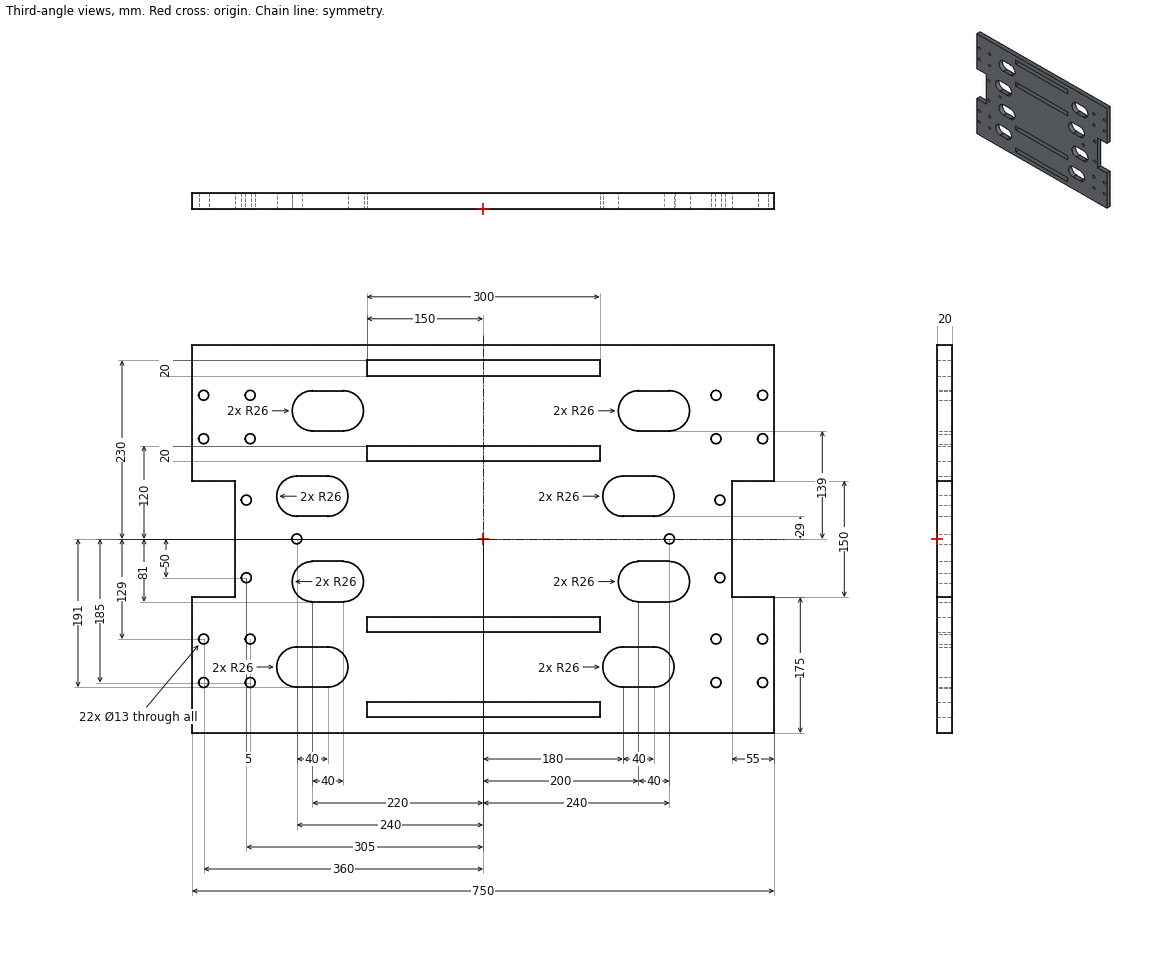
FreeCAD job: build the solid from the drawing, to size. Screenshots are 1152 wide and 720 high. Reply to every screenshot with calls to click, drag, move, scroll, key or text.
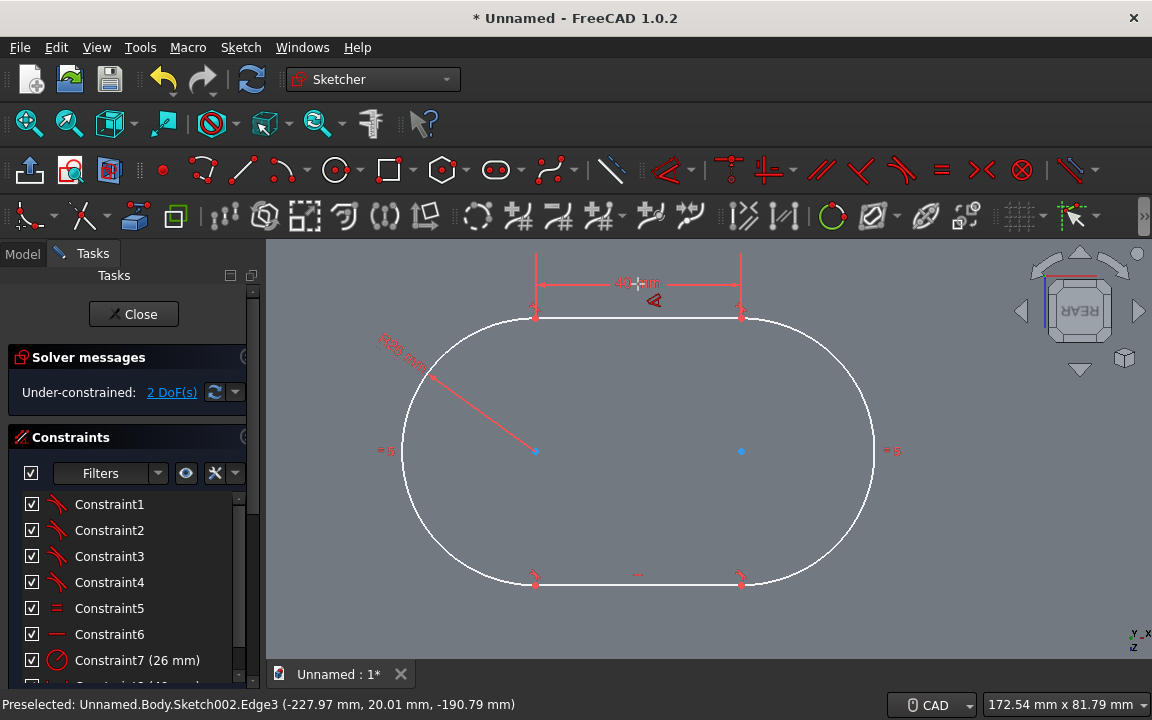
click(536, 318)
click(761, 284)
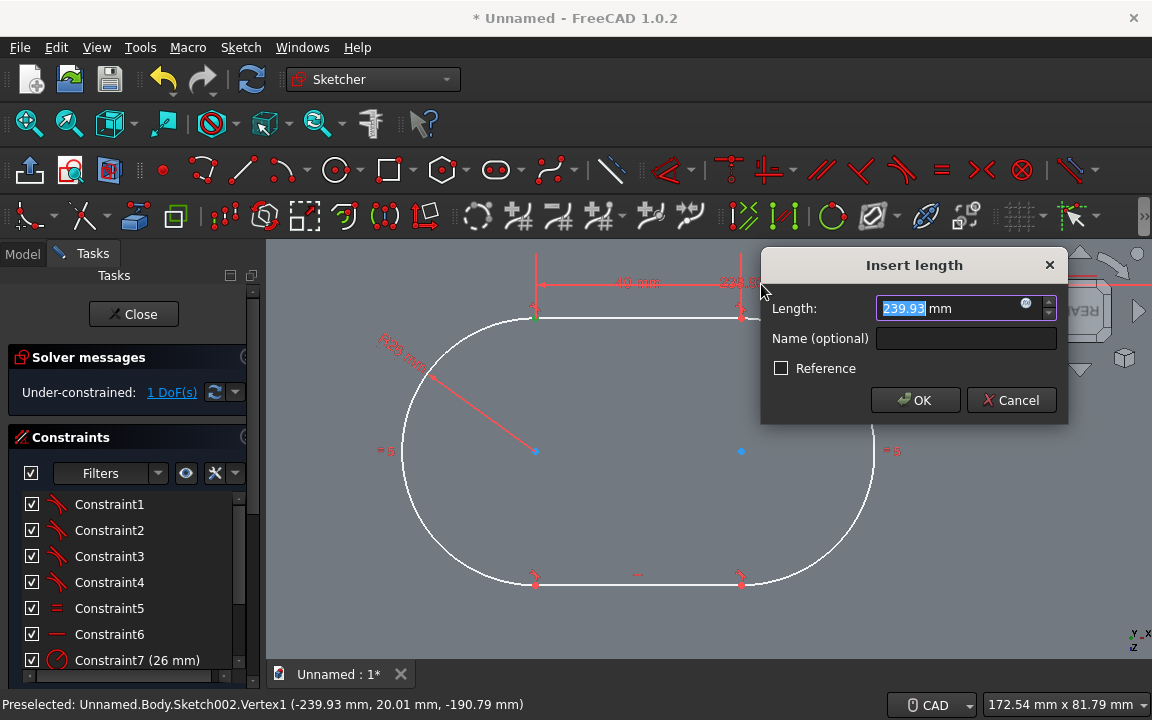
text(240)
key(Return)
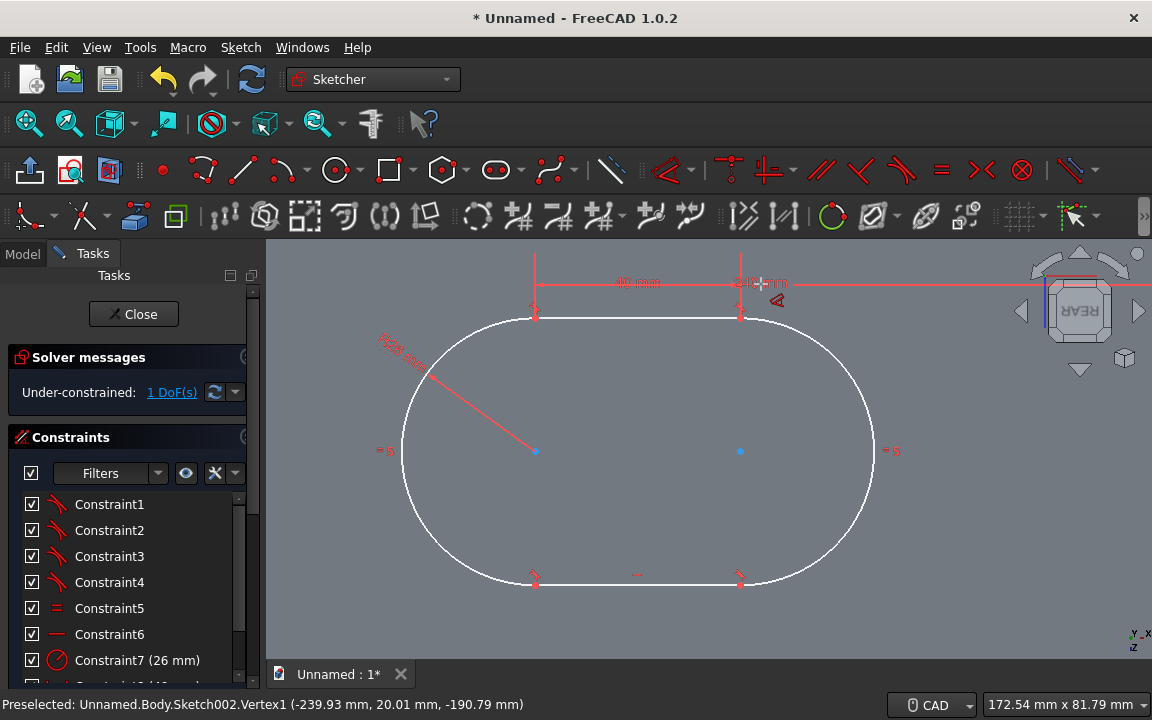
click(535, 318)
click(501, 475)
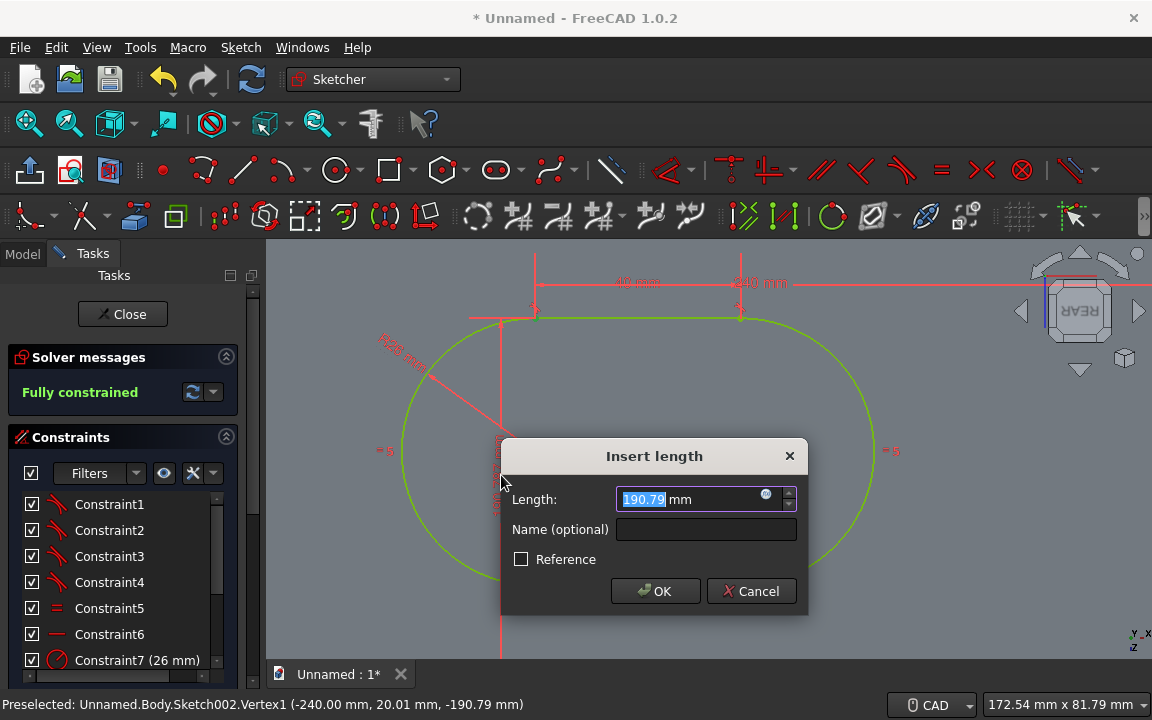
text(191)
key(Return)
key(Escape)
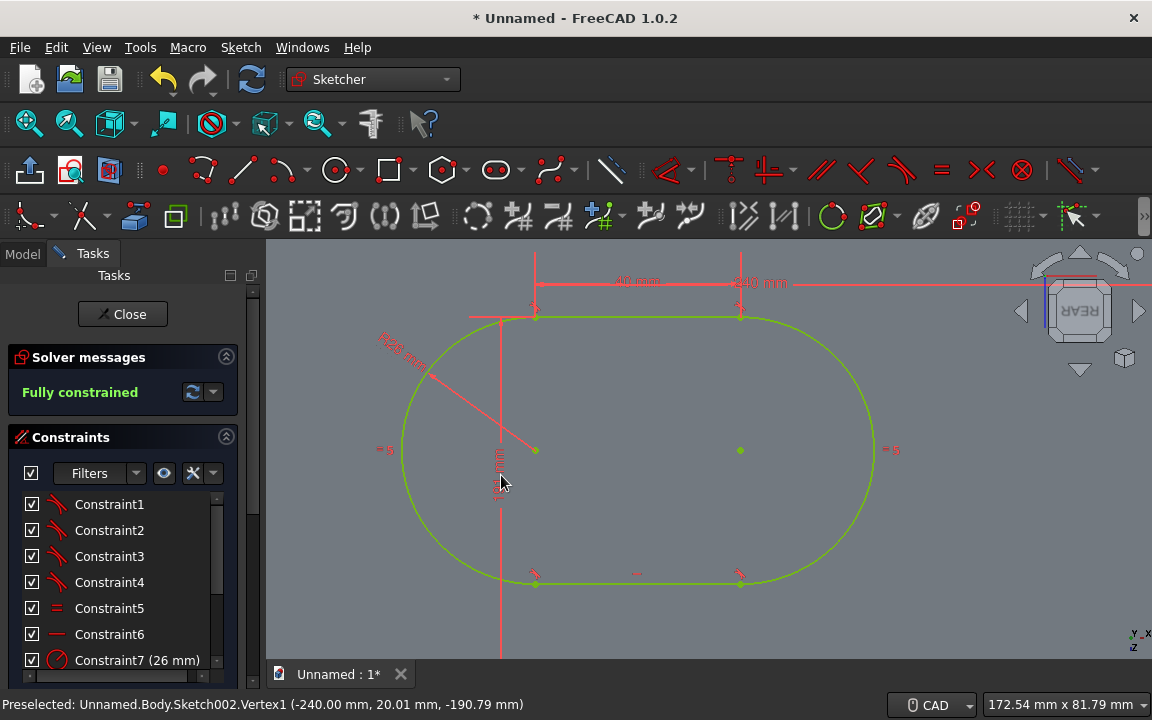
click(123, 314)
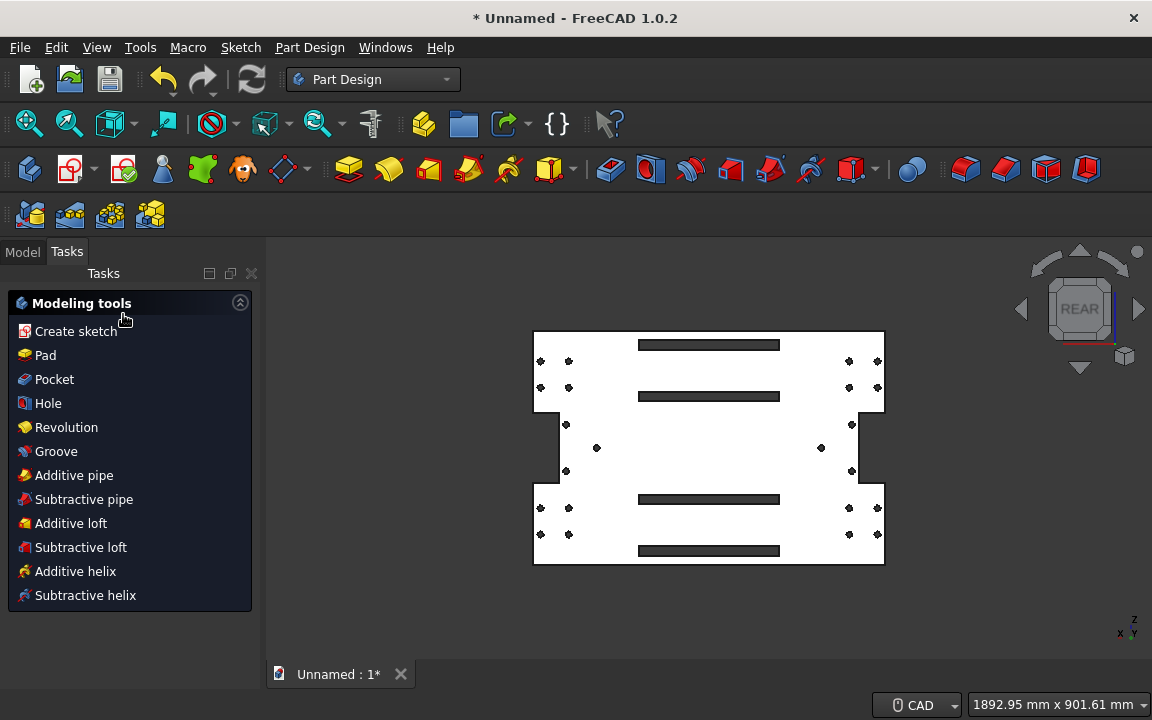
click(612, 170)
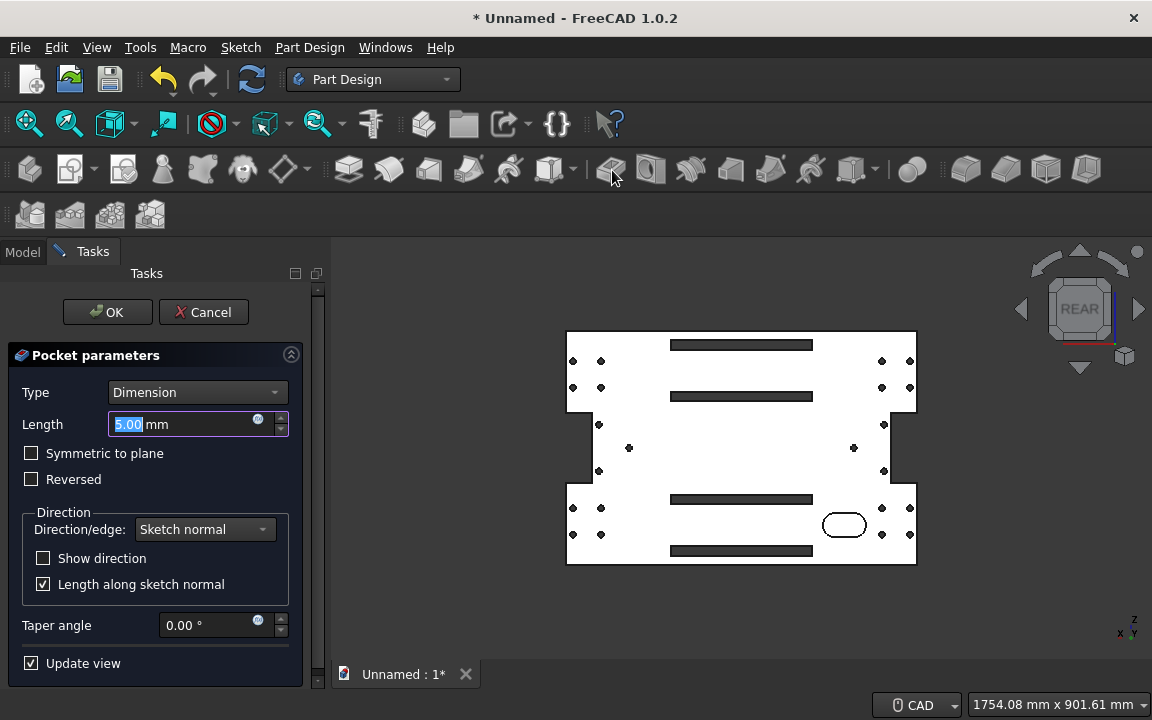
click(198, 392)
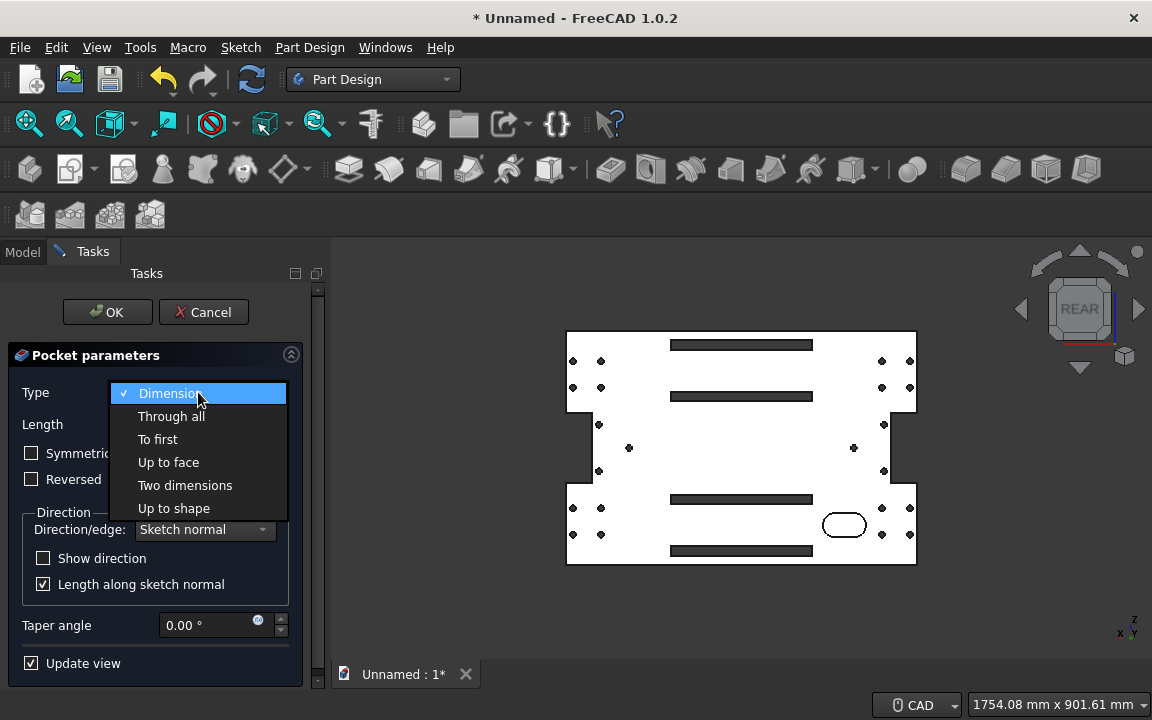
click(198, 440)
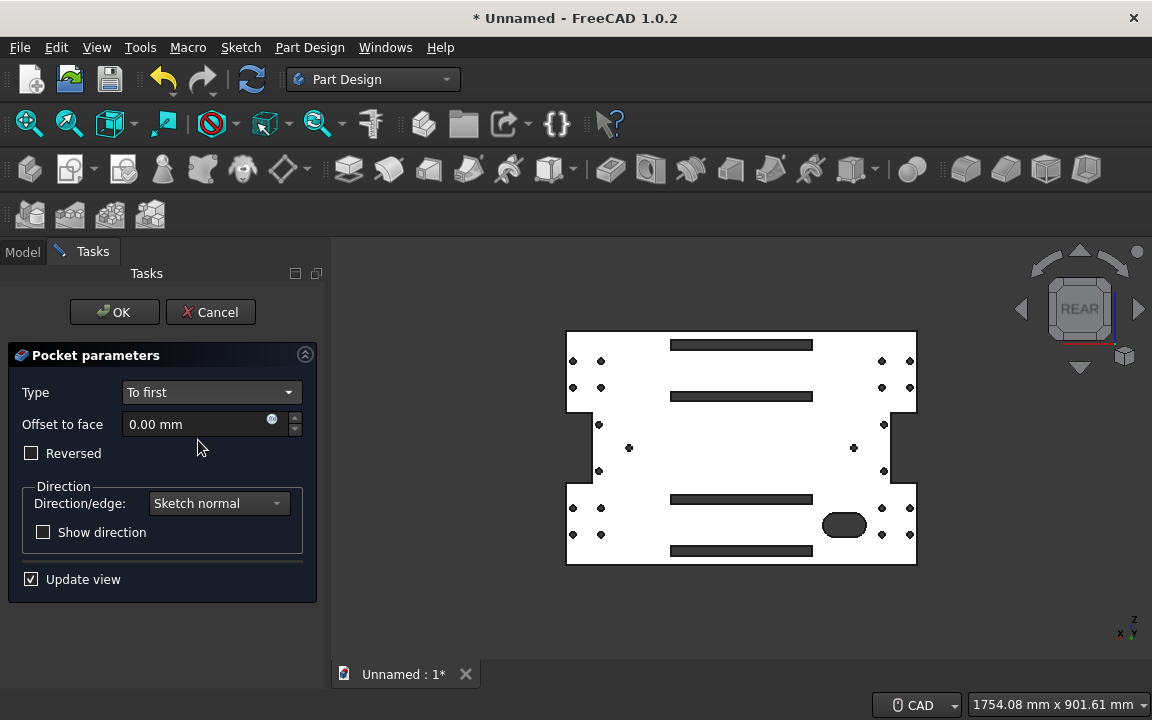
click(115, 312)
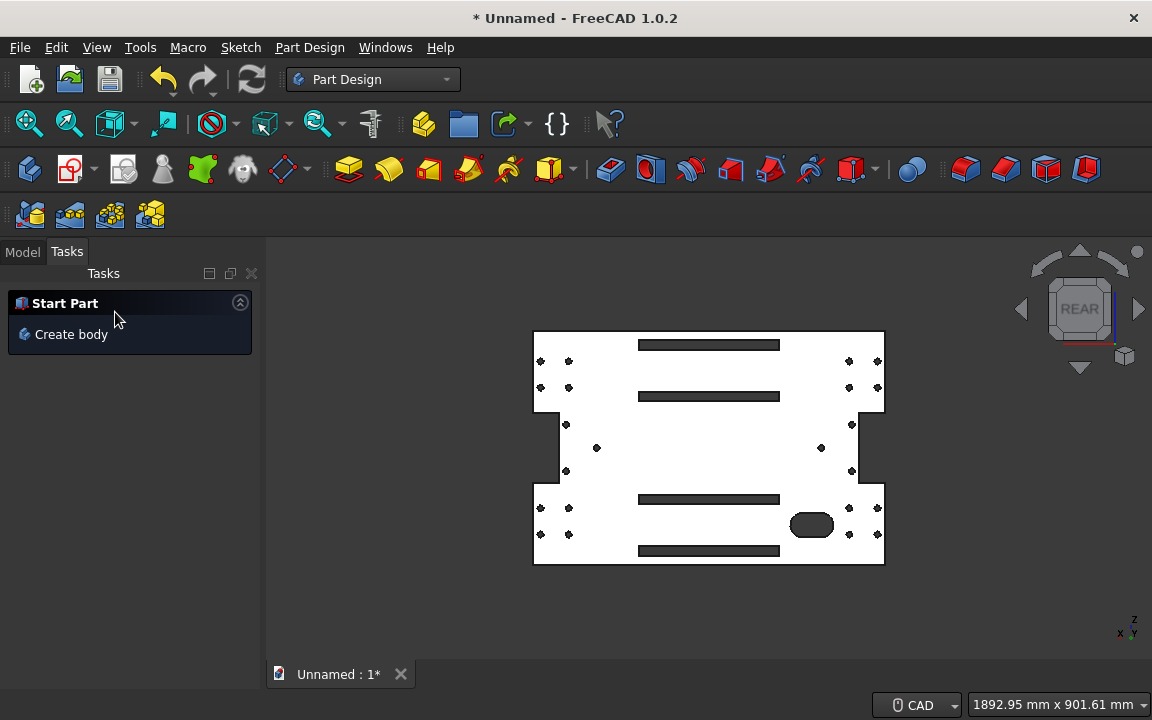
click(659, 447)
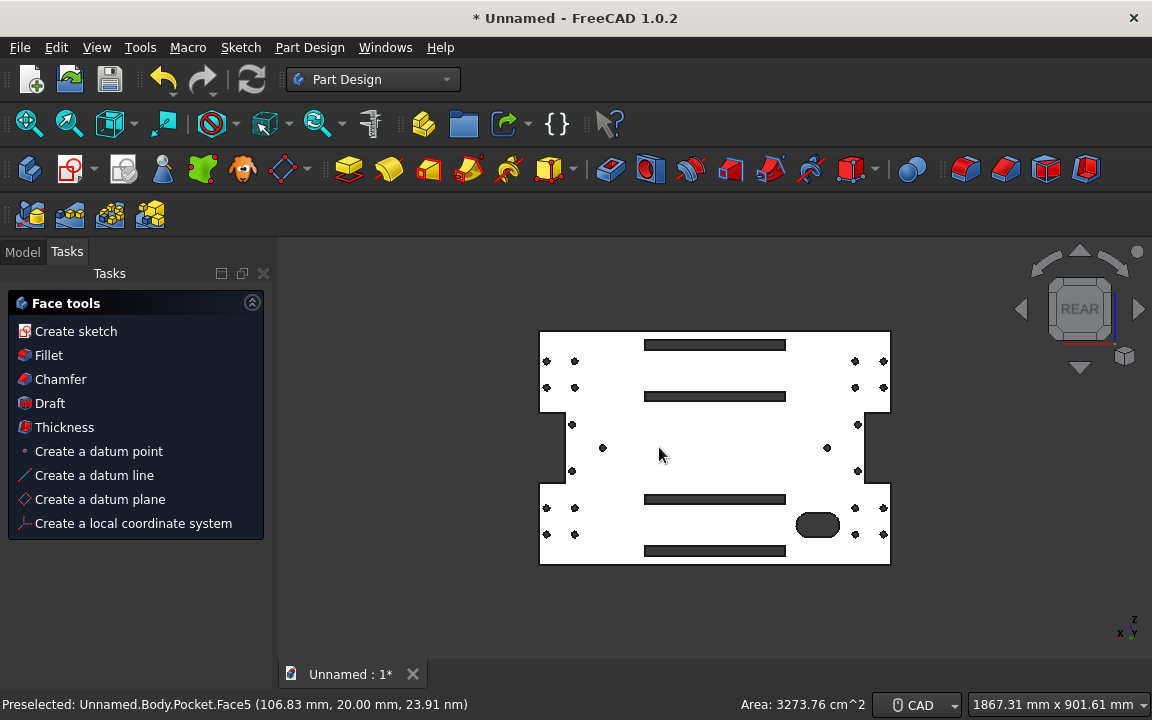
click(70, 170)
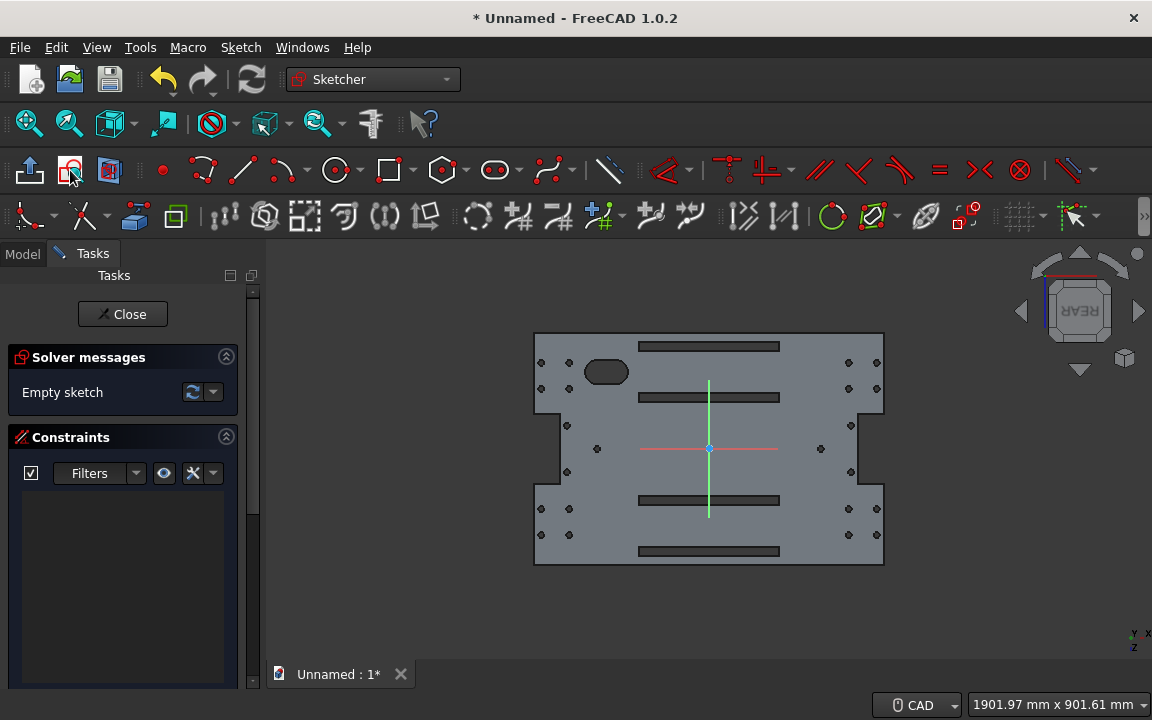
scroll(613, 421, up, 12)